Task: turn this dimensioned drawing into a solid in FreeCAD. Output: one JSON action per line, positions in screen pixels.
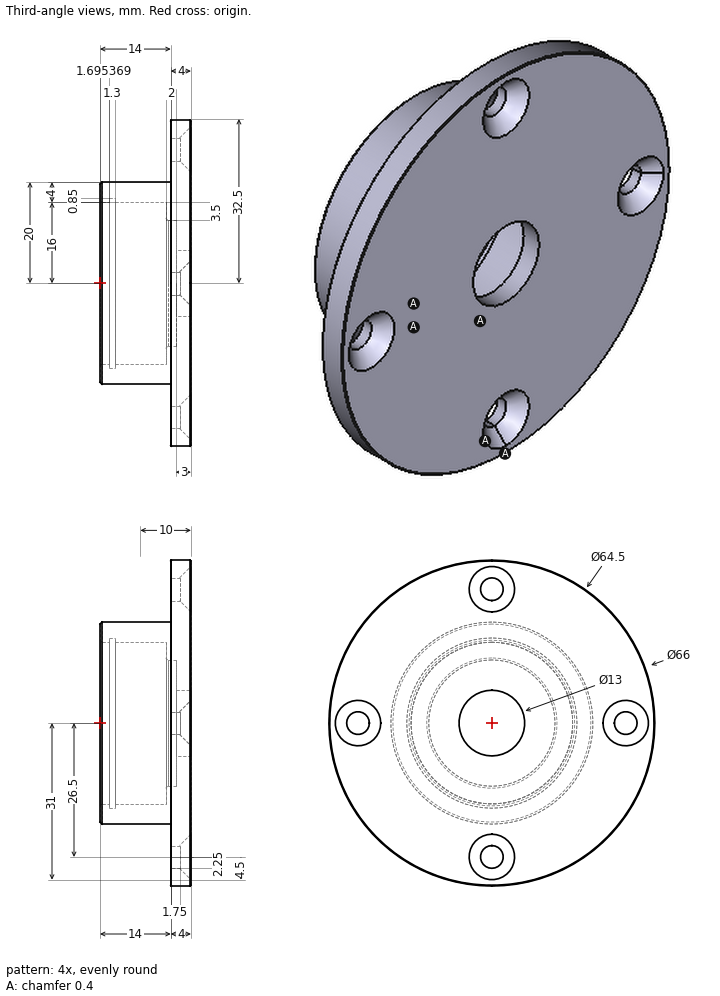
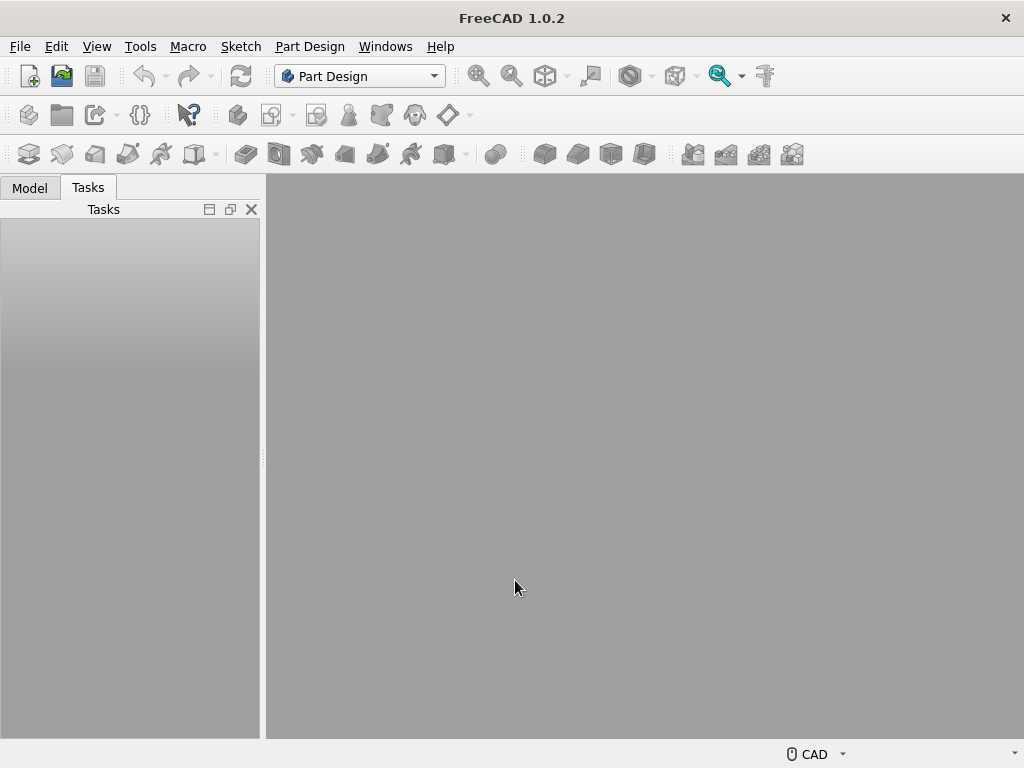
{"action": "left_click", "coordinate": [29, 76]}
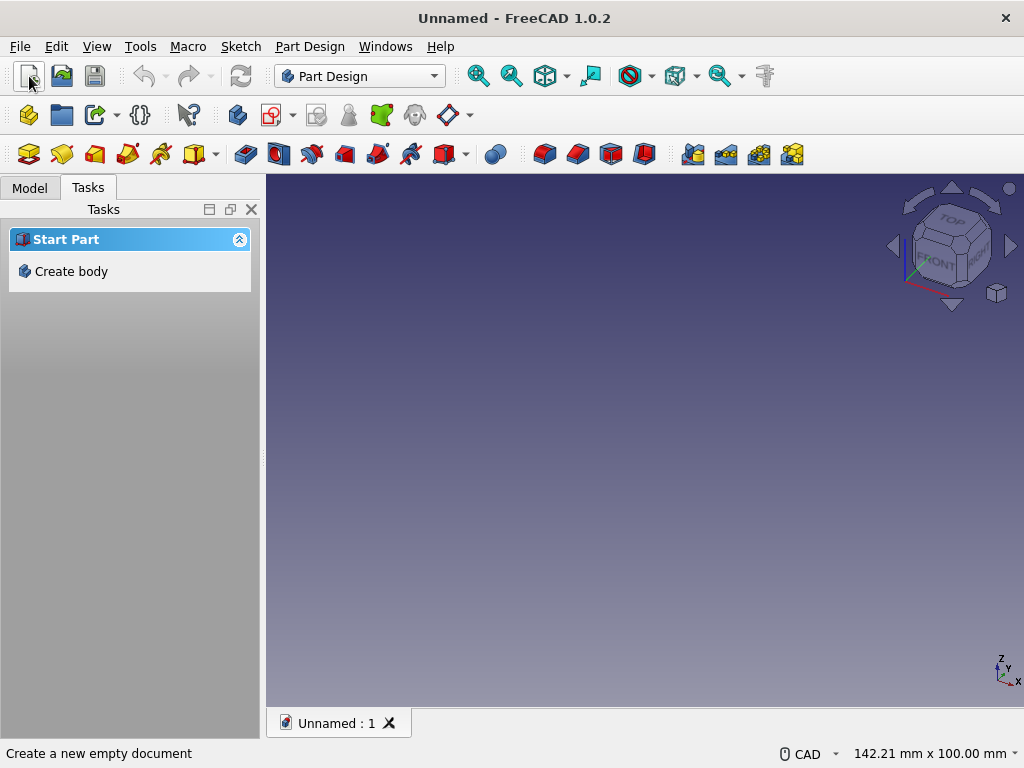
{"action": "left_click", "coordinate": [270, 116]}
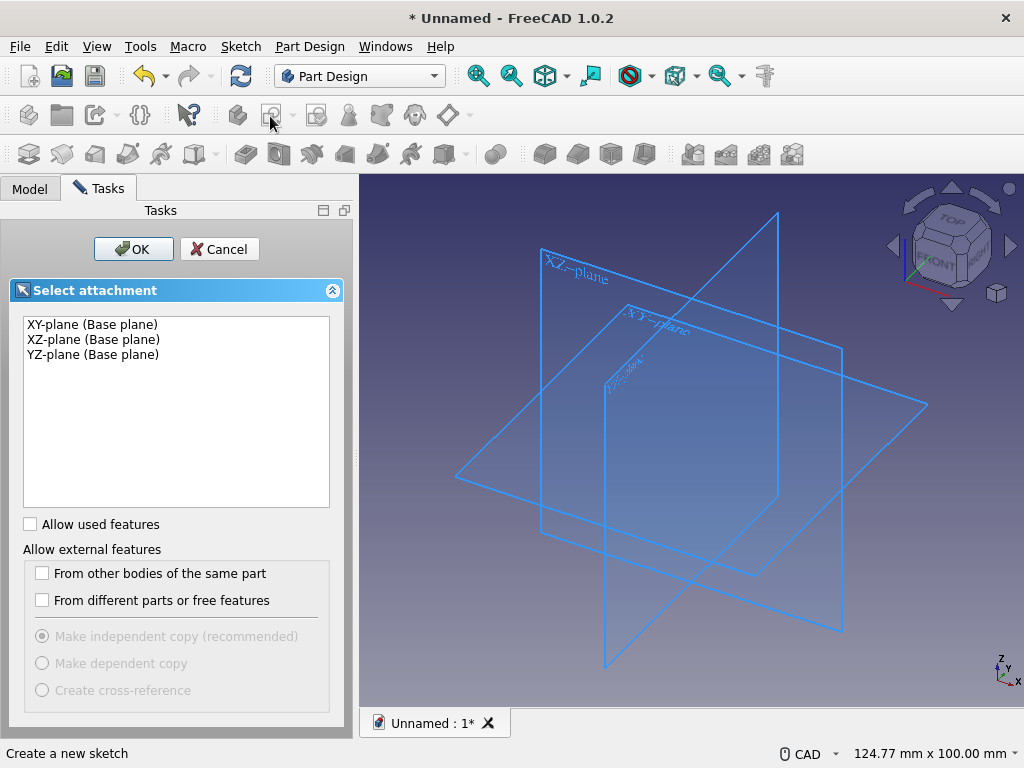
{"action": "left_click", "coordinate": [84, 324]}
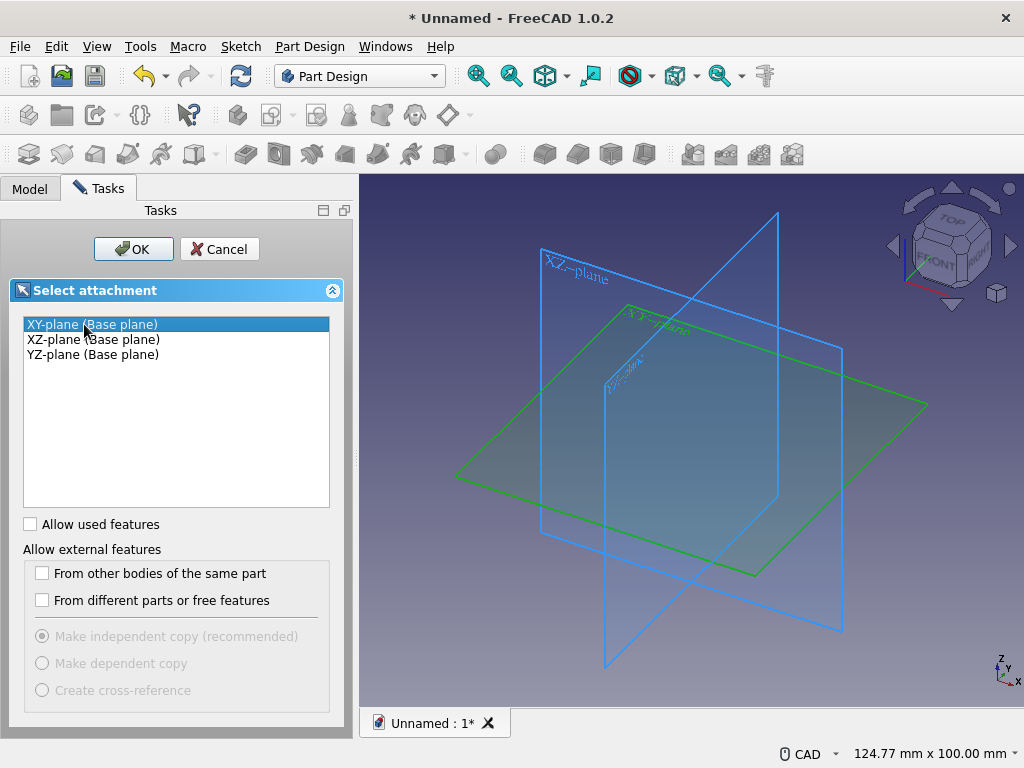
{"action": "left_click", "coordinate": [134, 249]}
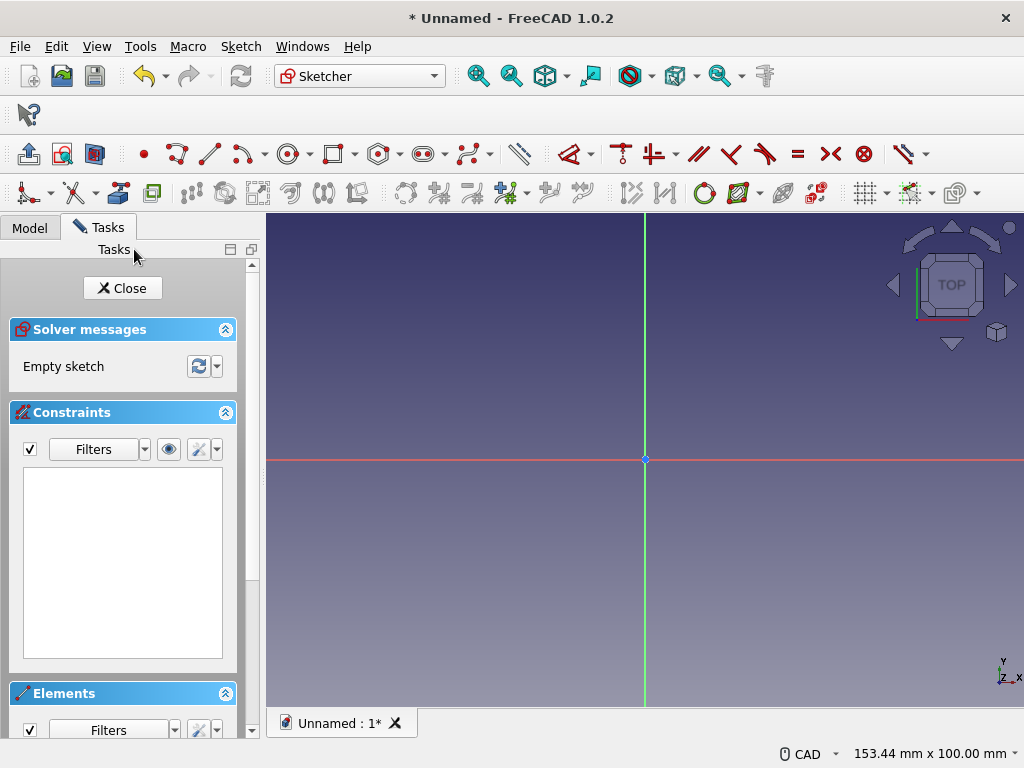
{"action": "scroll", "coordinate": [827, 282], "scroll_direction": "up", "scroll_amount": 3}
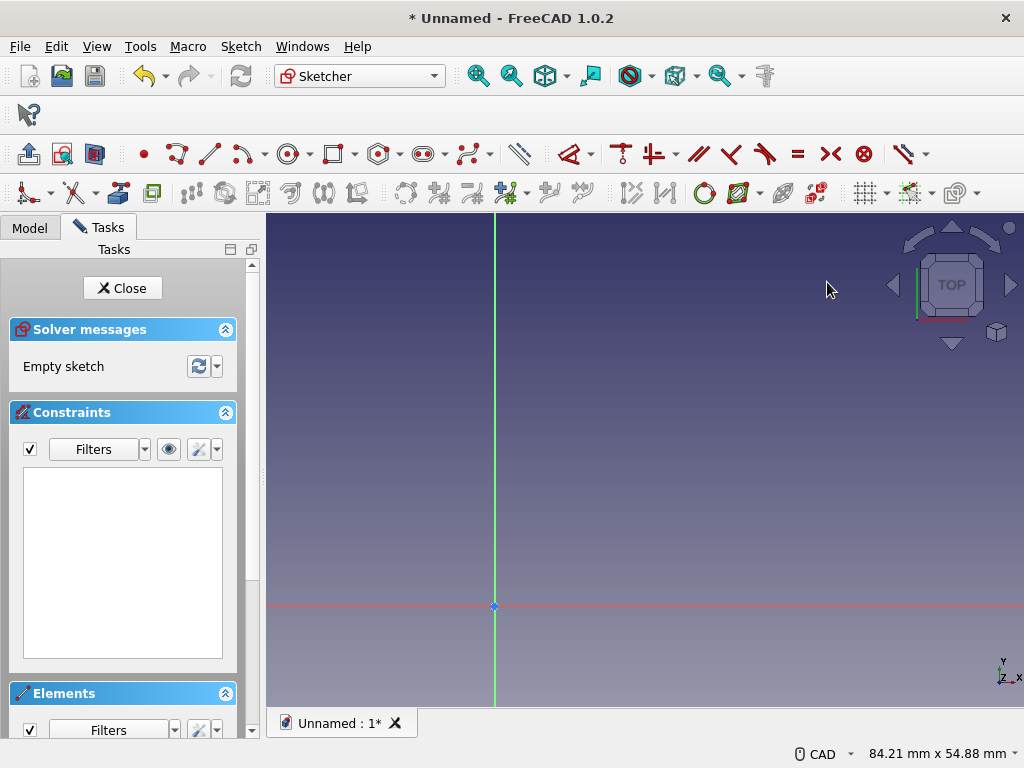
{"action": "left_click", "coordinate": [177, 154]}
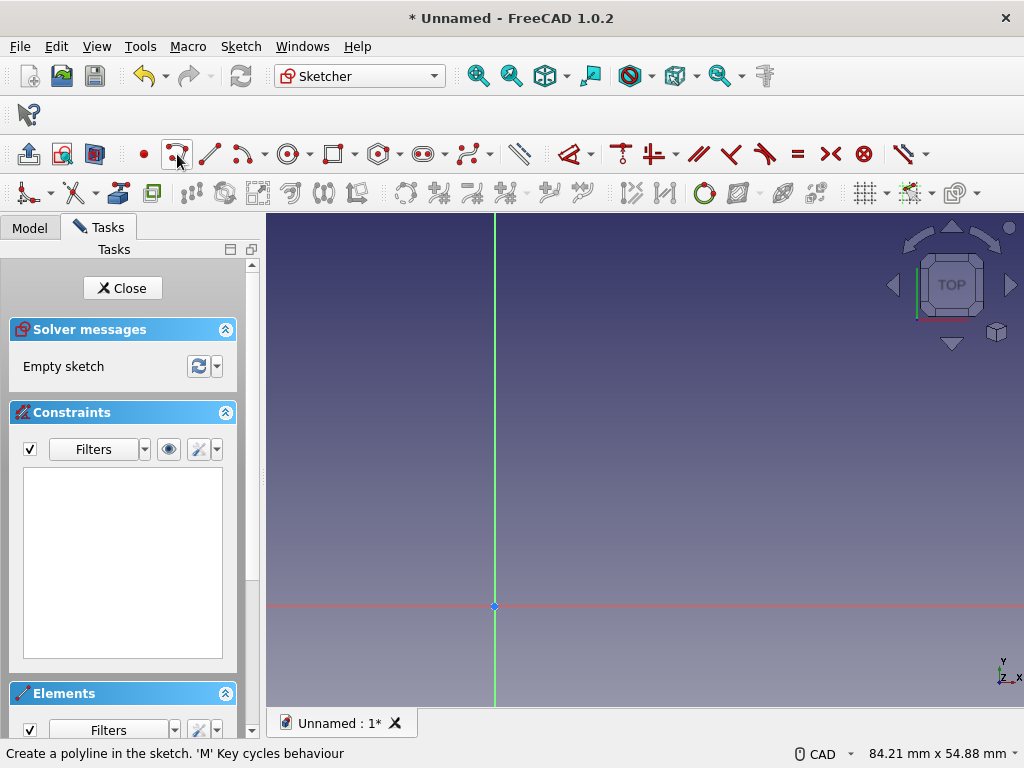
{"action": "left_click", "coordinate": [630, 606]}
{"action": "left_click", "coordinate": [657, 597]}
{"action": "left_click", "coordinate": [657, 314]}
{"action": "left_click", "coordinate": [621, 314]}
{"action": "left_click", "coordinate": [621, 426]}
{"action": "left_click", "coordinate": [495, 426]}
{"action": "left_click", "coordinate": [504, 462]}
{"action": "left_click", "coordinate": [510, 462]}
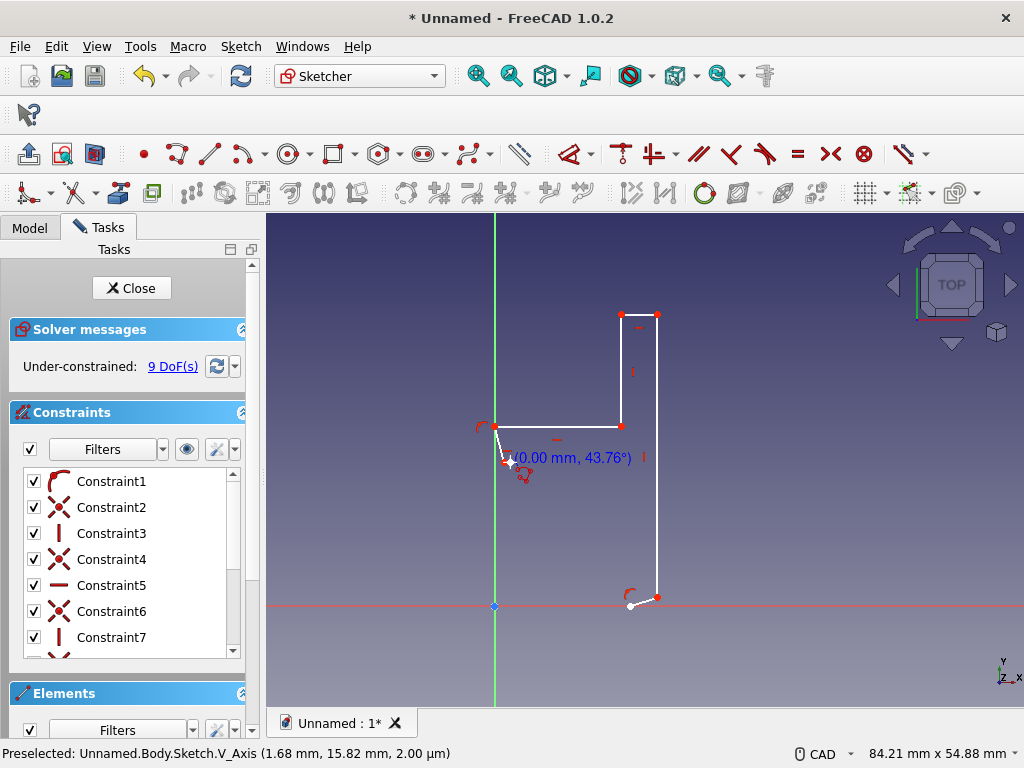
{"action": "scroll", "coordinate": [510, 455], "scroll_direction": "up", "scroll_amount": 4}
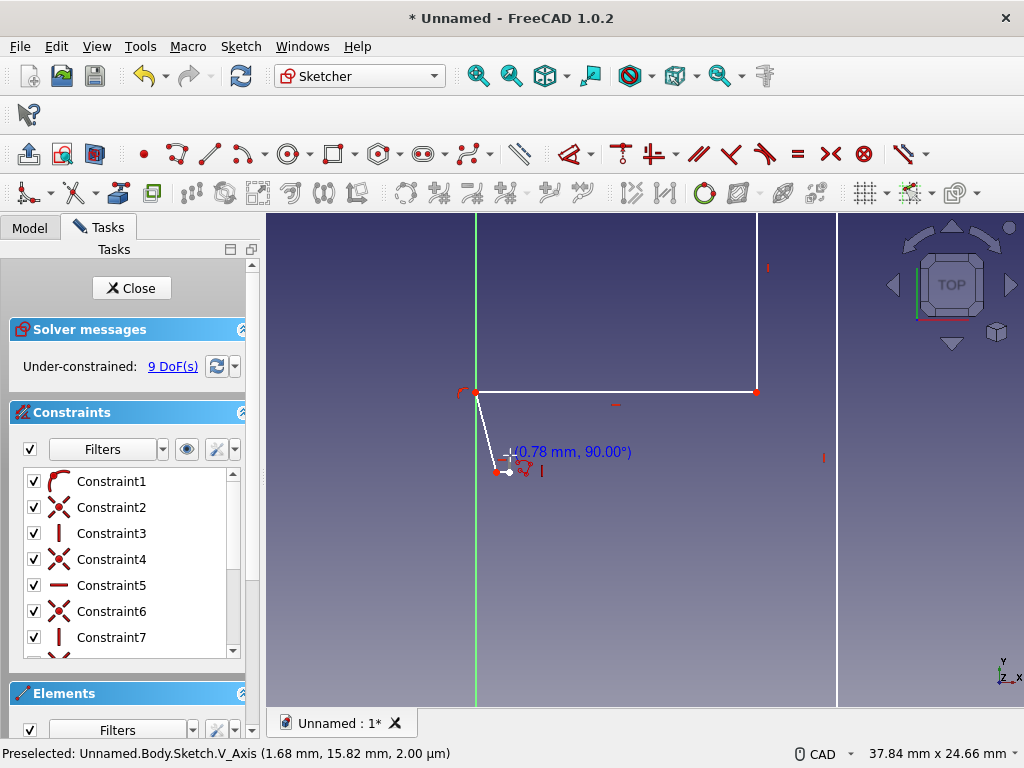
{"action": "left_click", "coordinate": [510, 453]}
{"action": "left_click", "coordinate": [536, 453]}
{"action": "left_click", "coordinate": [536, 470]}
{"action": "left_click", "coordinate": [736, 470]}
{"action": "left_click", "coordinate": [736, 541]}
{"action": "left_click", "coordinate": [776, 541]}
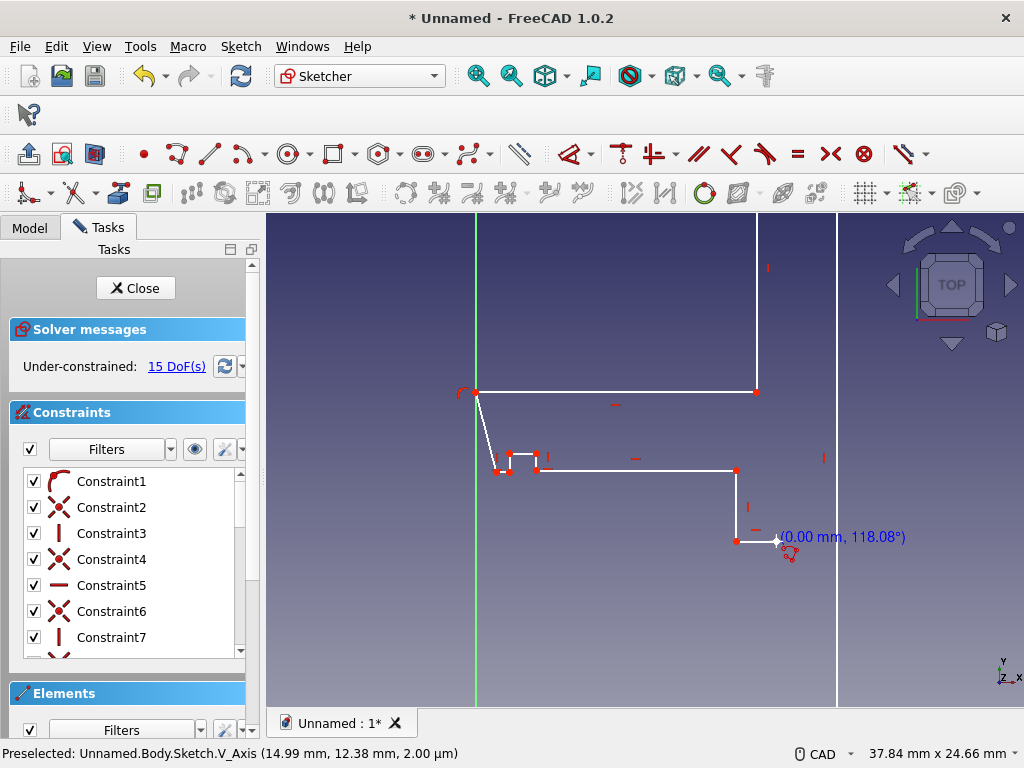
{"action": "scroll", "coordinate": [512, 456], "scroll_direction": "down", "scroll_amount": 4}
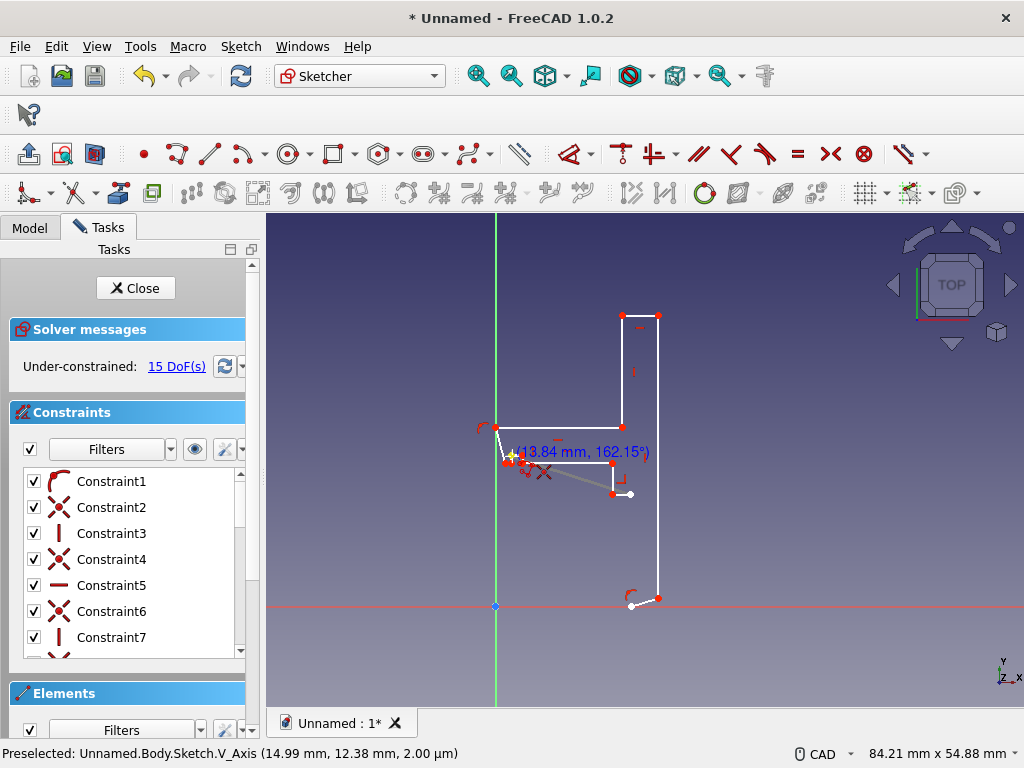
{"action": "left_click", "coordinate": [631, 607]}
{"action": "key", "text": "Escape"}
{"action": "key", "text": "Escape"}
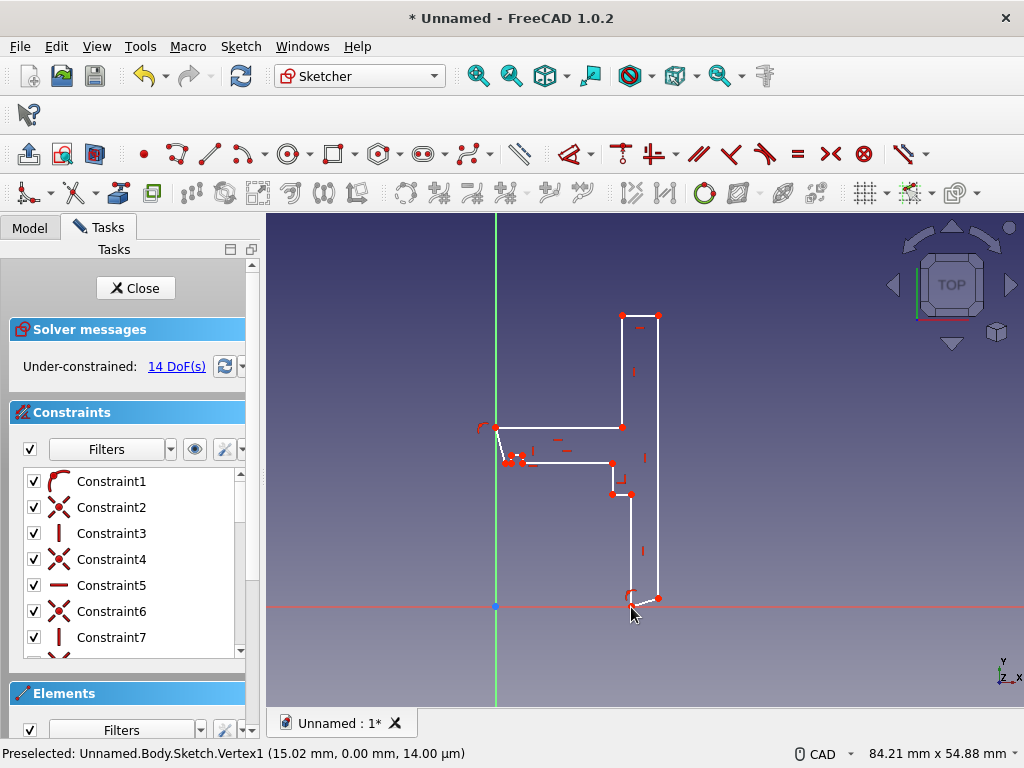
{"action": "scroll", "coordinate": [642, 603], "scroll_direction": "up", "scroll_amount": 2}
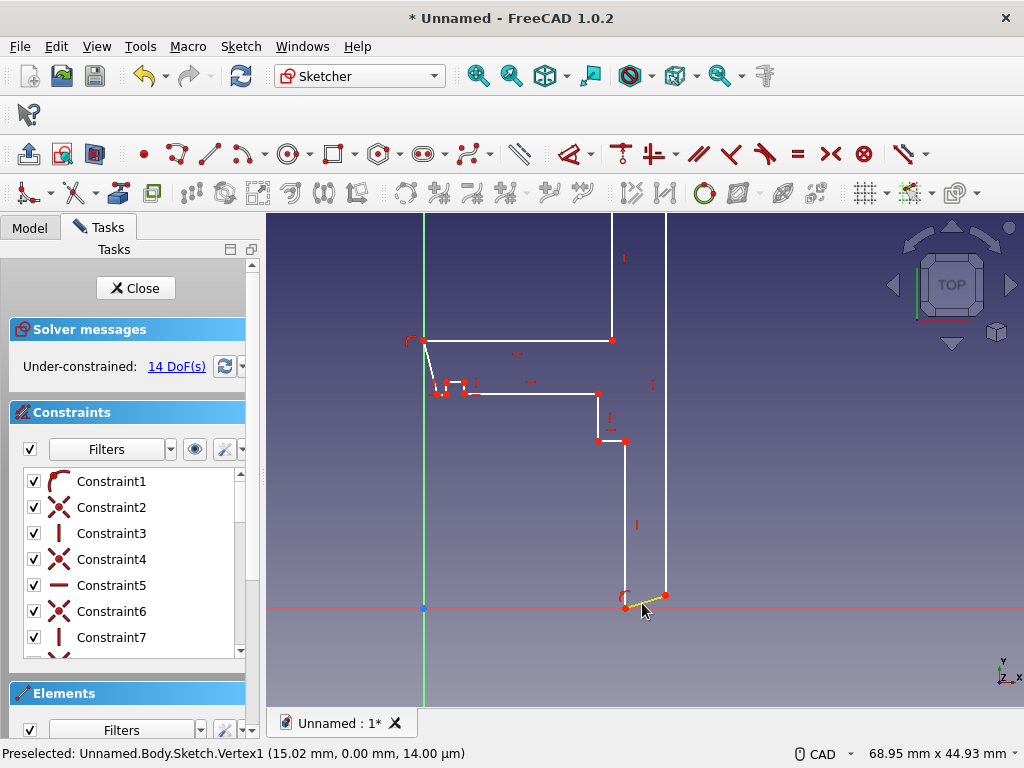
{"action": "left_click", "coordinate": [642, 603]}